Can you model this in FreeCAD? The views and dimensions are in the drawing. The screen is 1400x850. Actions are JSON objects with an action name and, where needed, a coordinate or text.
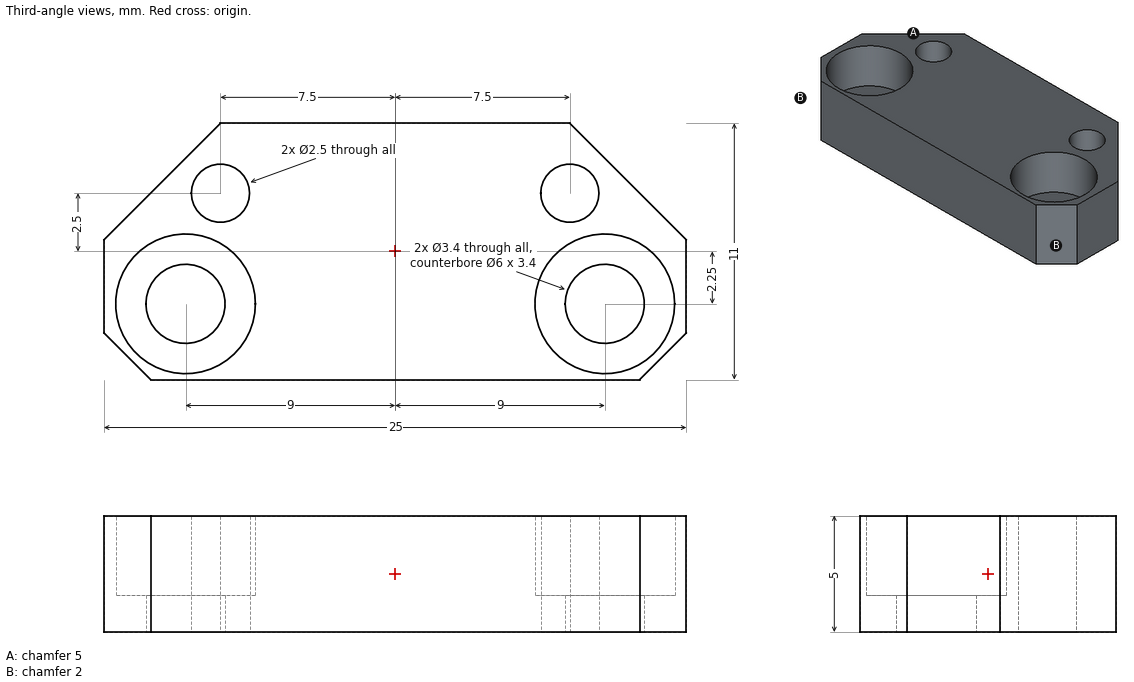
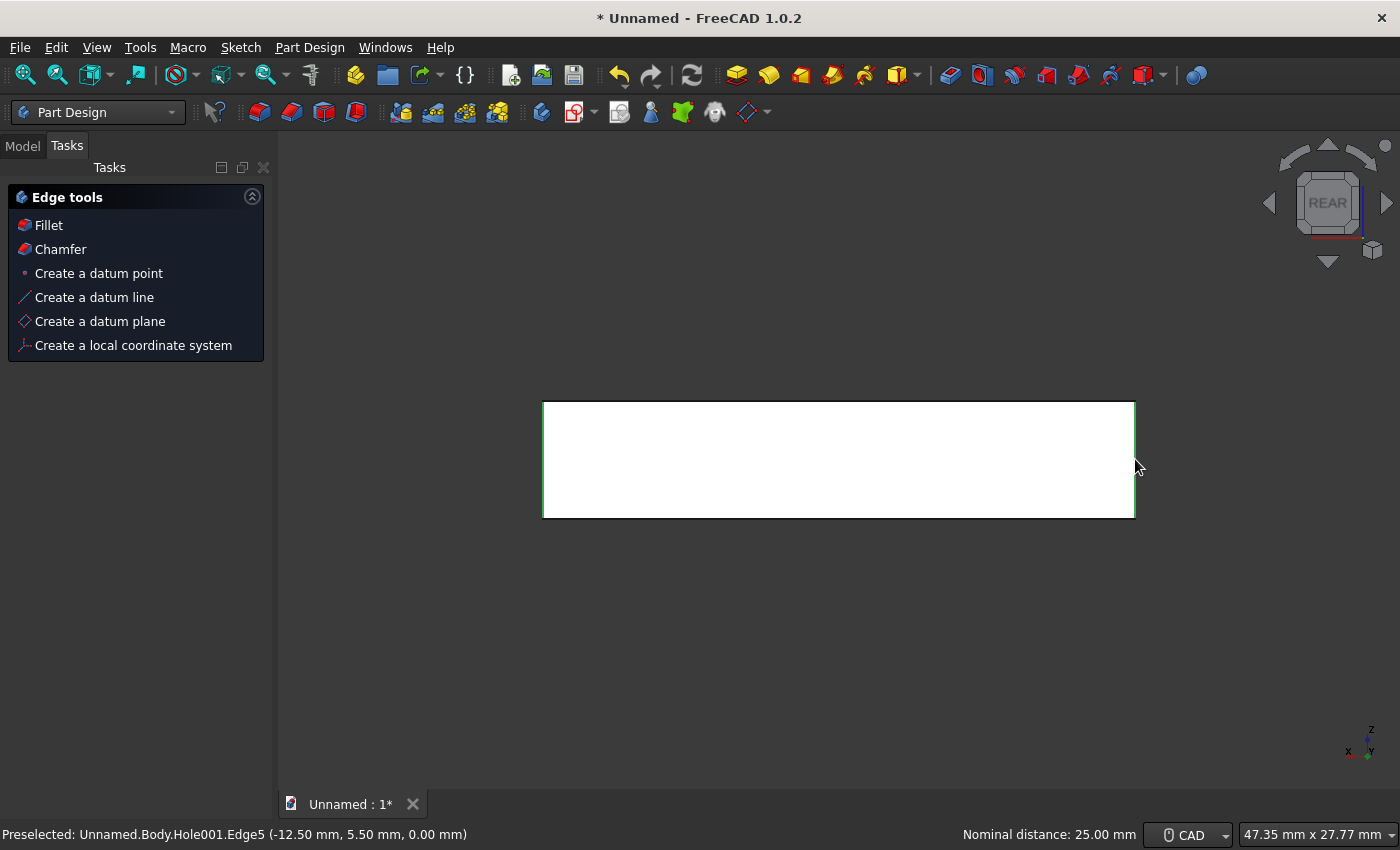
{"action": "left_click", "coordinate": [292, 112]}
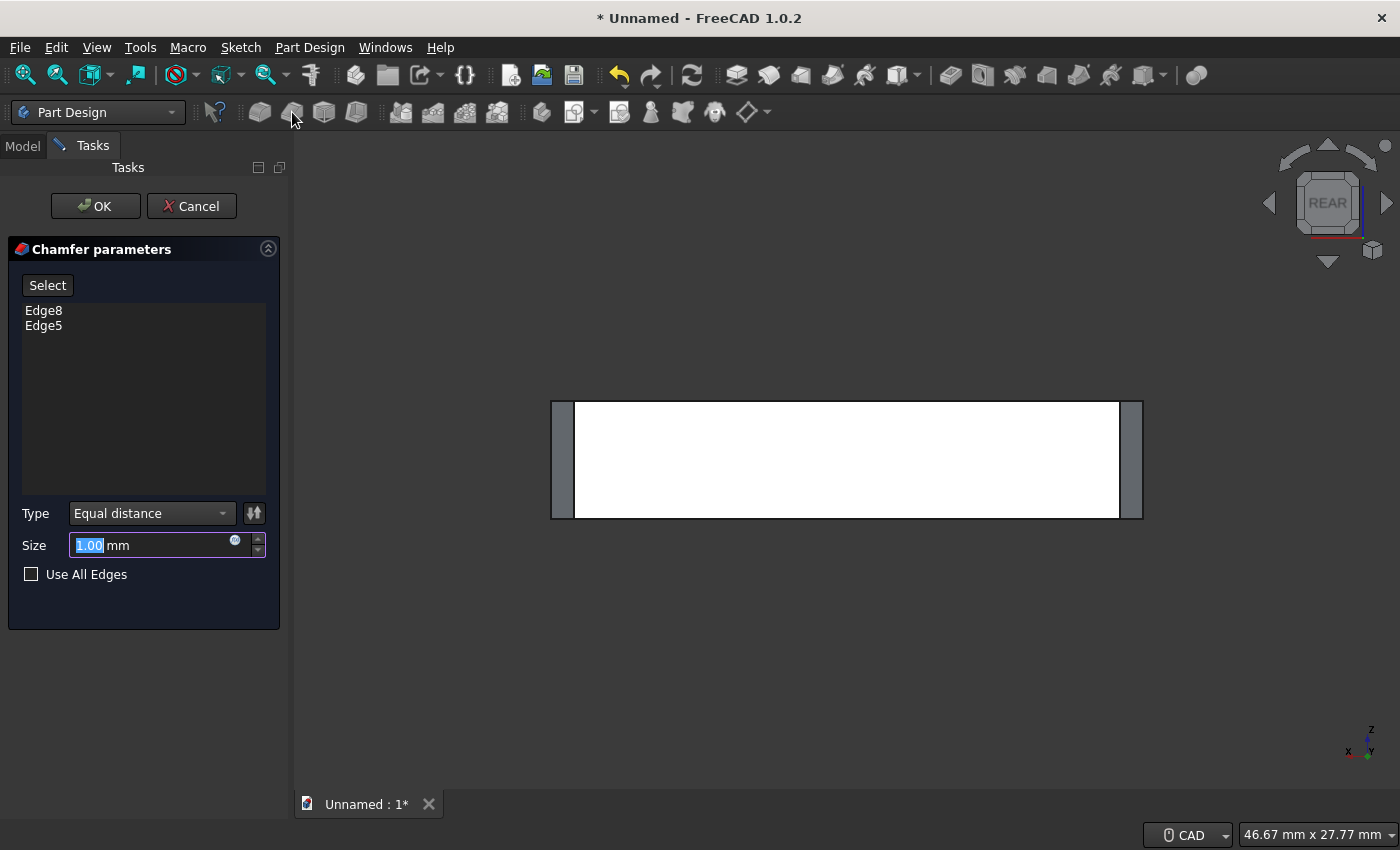
{"action": "type", "text": "5"}
{"action": "key", "text": "Tab"}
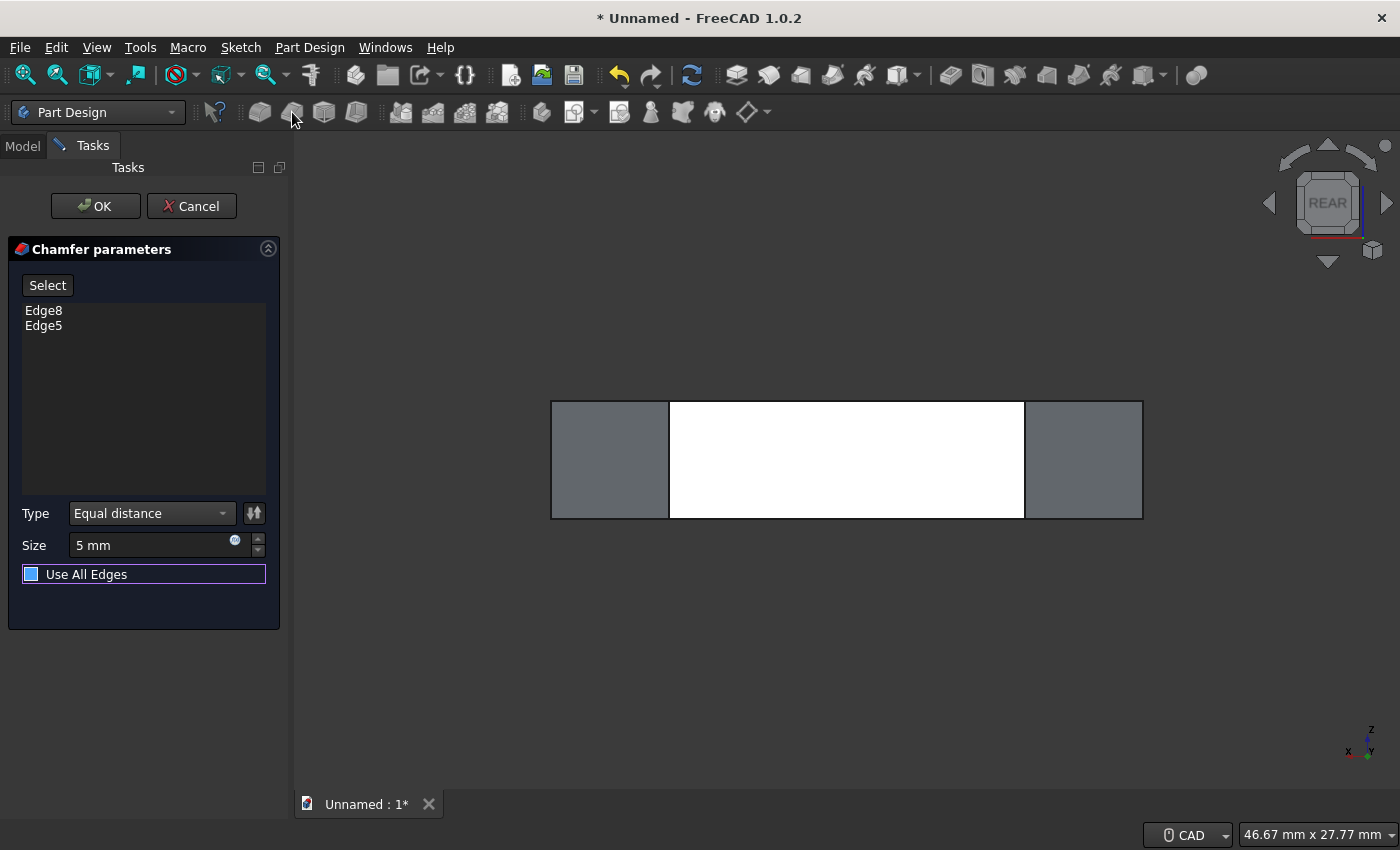
{"action": "left_click", "coordinate": [96, 206]}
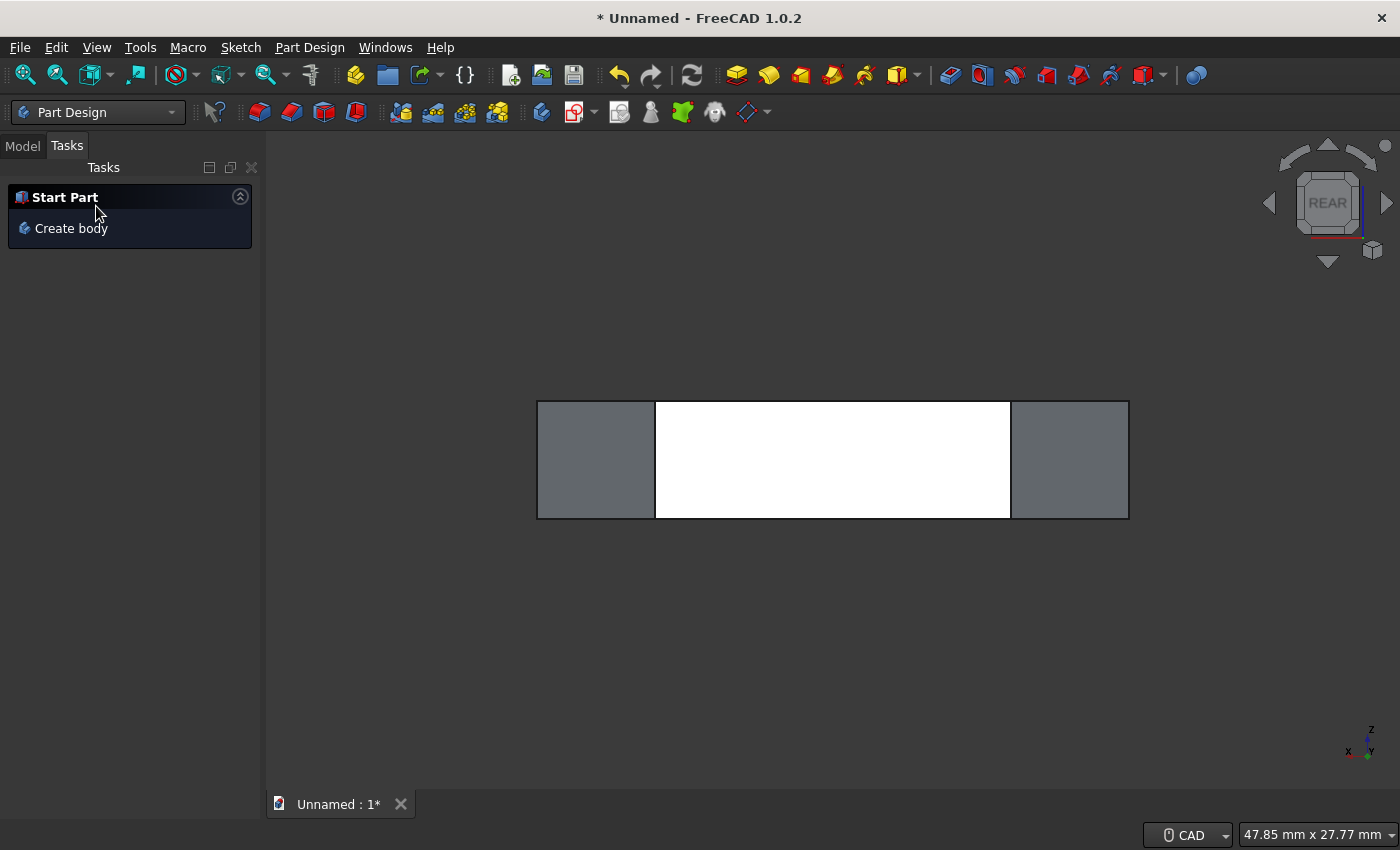
{"action": "key", "text": "0"}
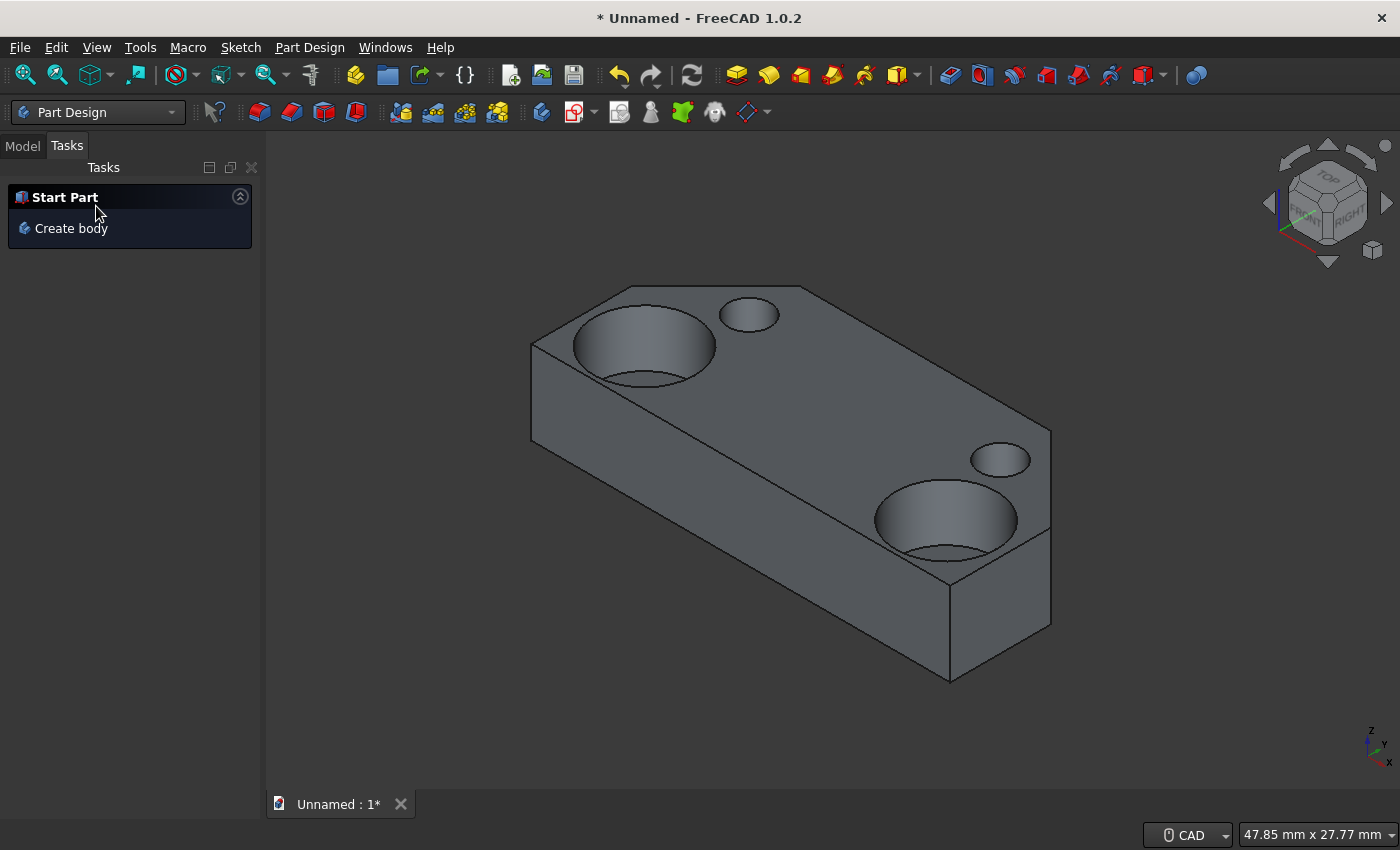
{"action": "left_click", "coordinate": [950, 633]}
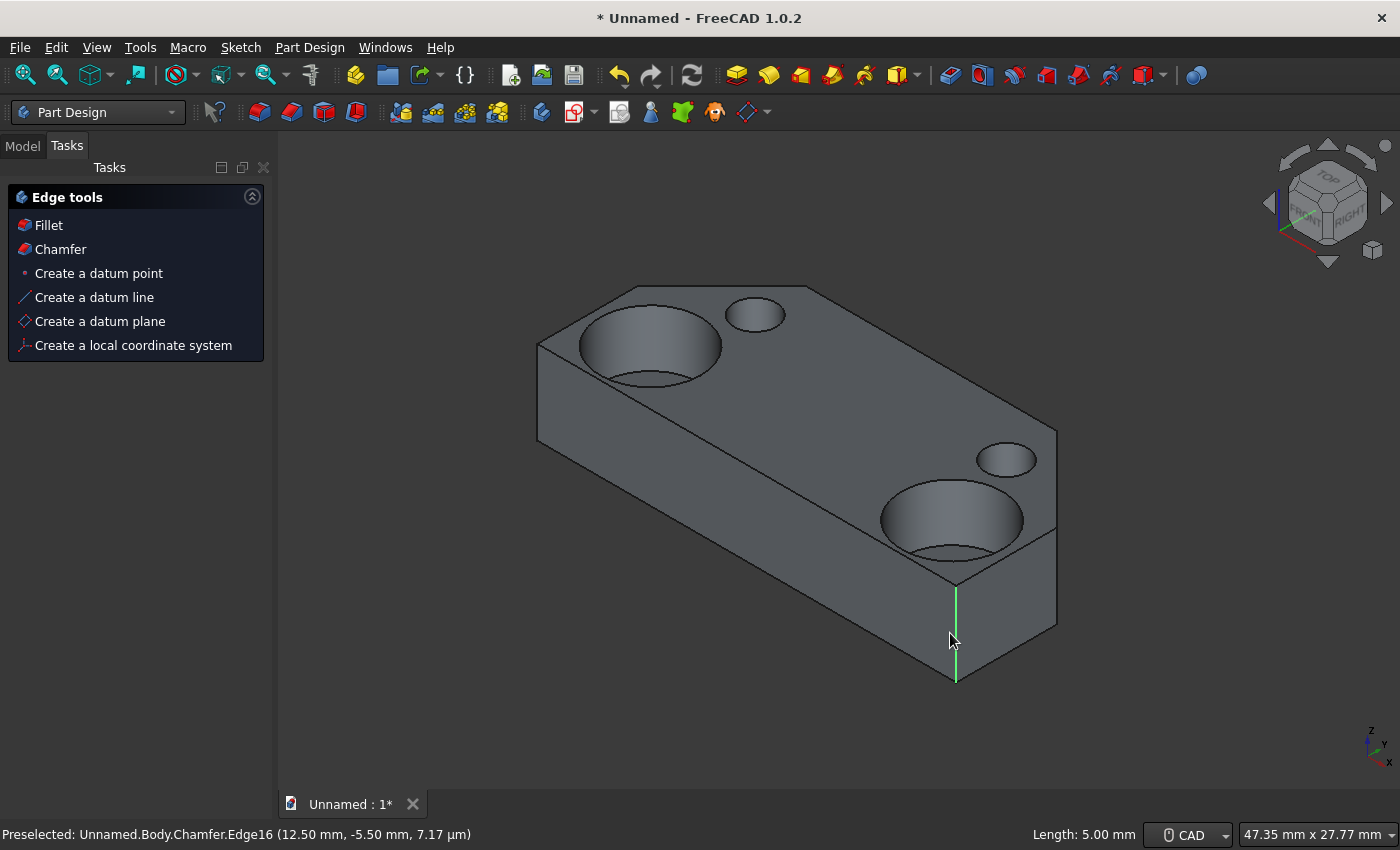
{"action": "key", "text": "2"}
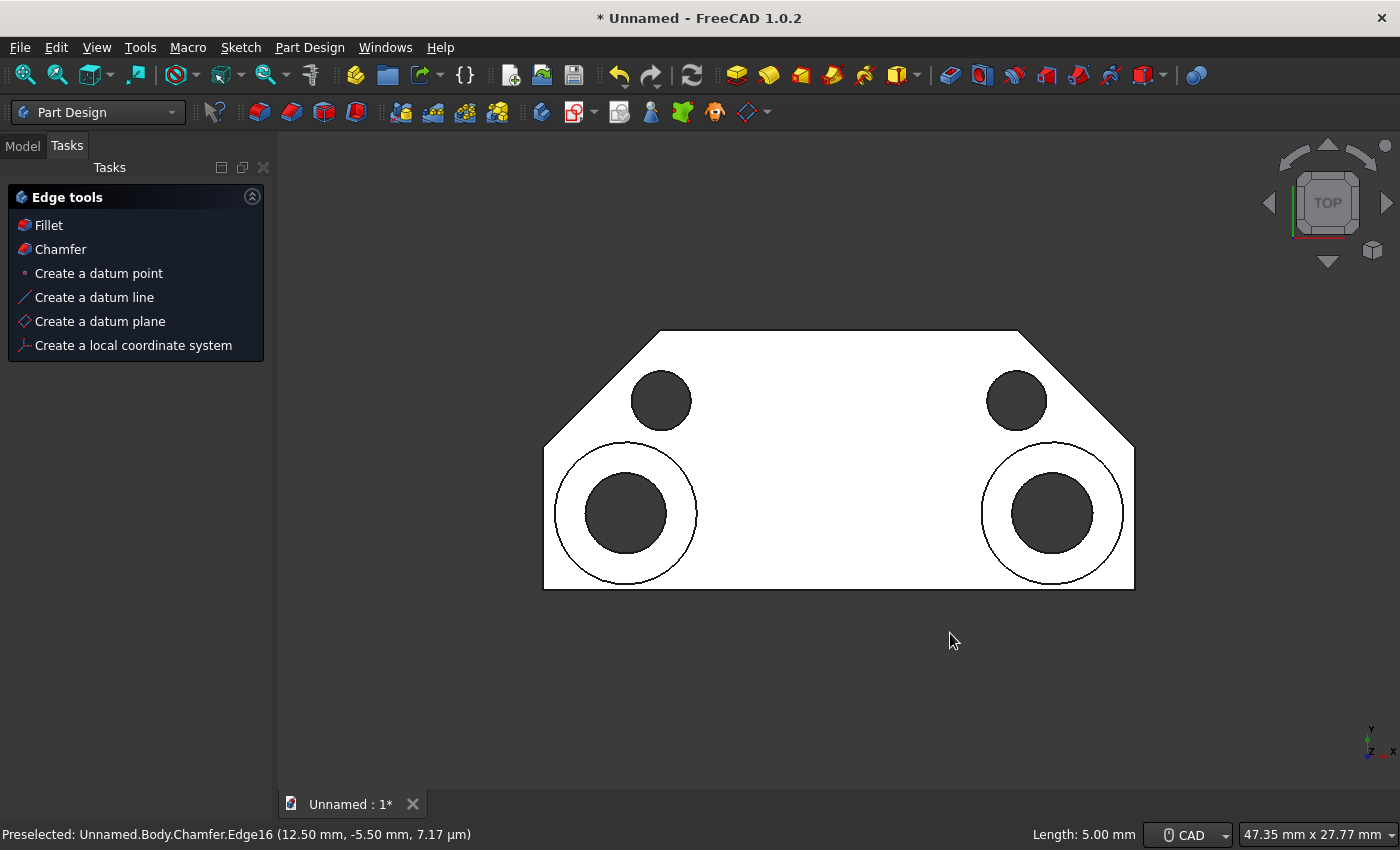
{"action": "key", "text": "1"}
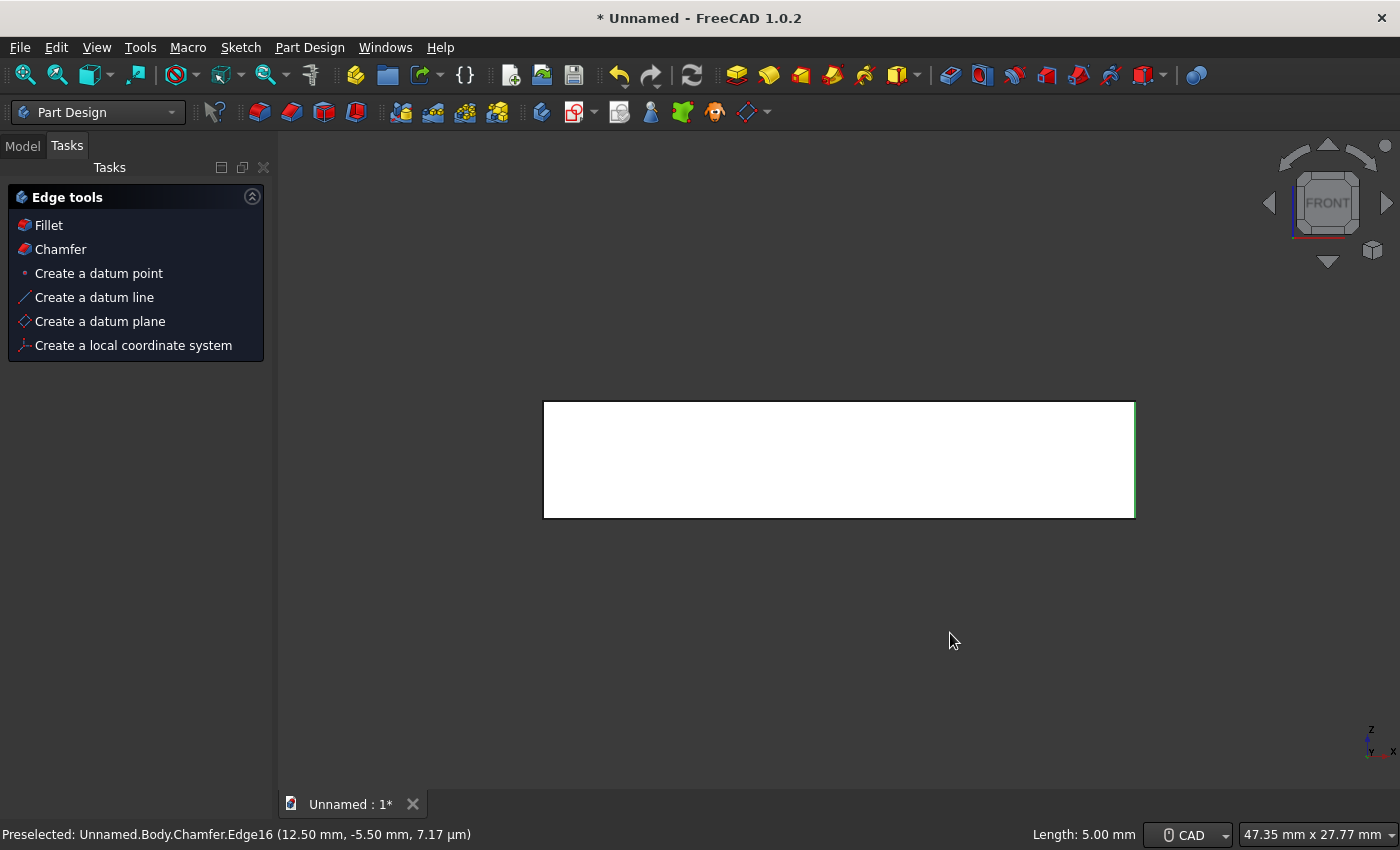
{"action": "left_click", "coordinate": [543, 459], "text": "ctrl"}